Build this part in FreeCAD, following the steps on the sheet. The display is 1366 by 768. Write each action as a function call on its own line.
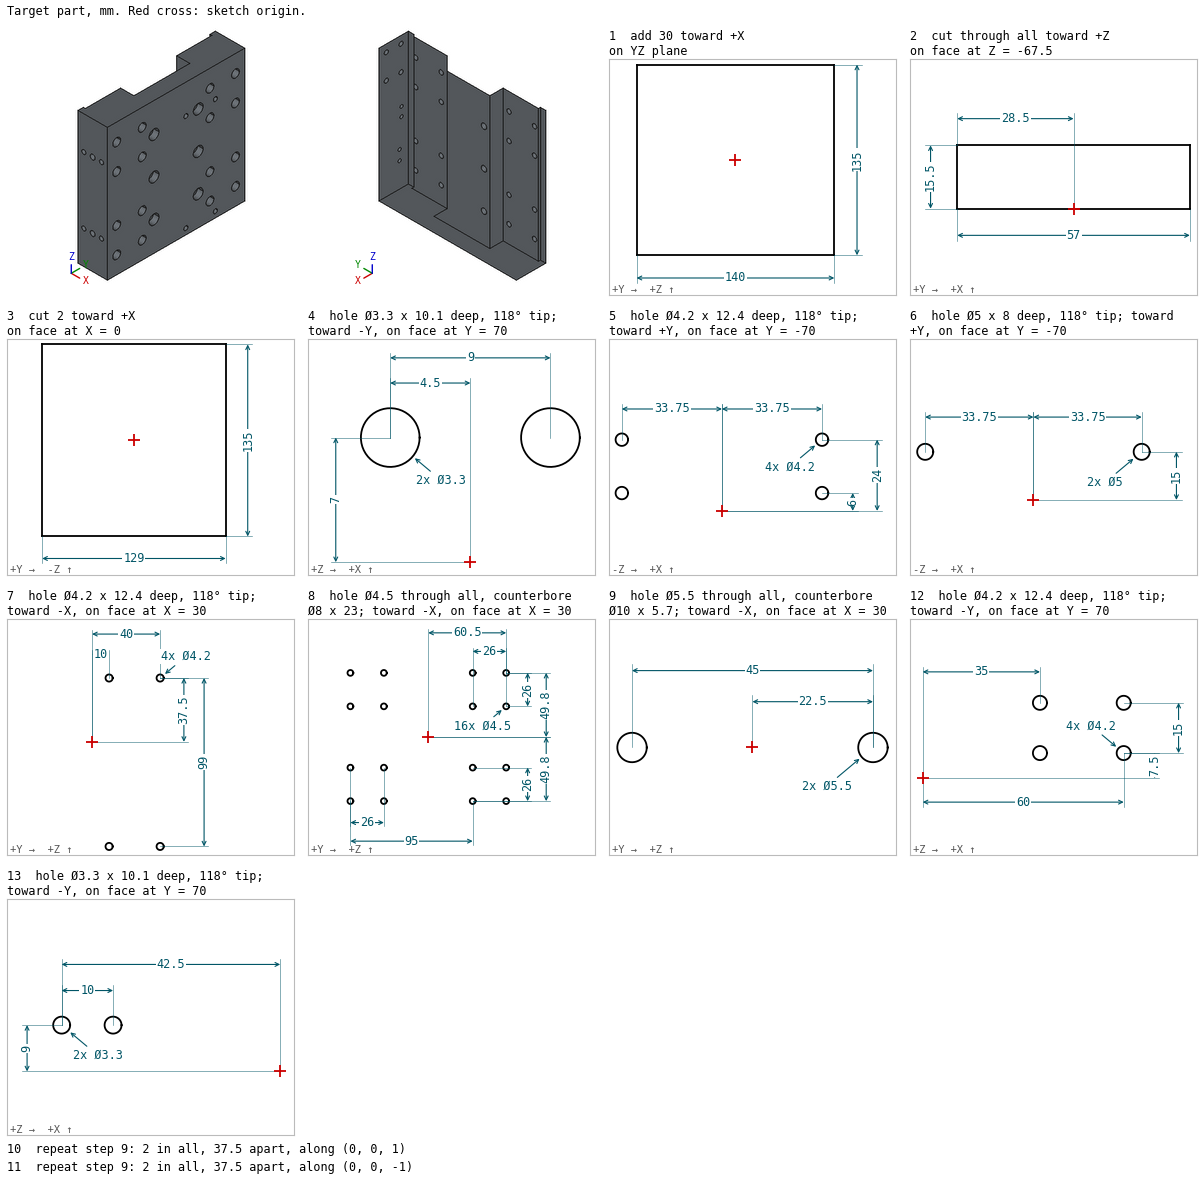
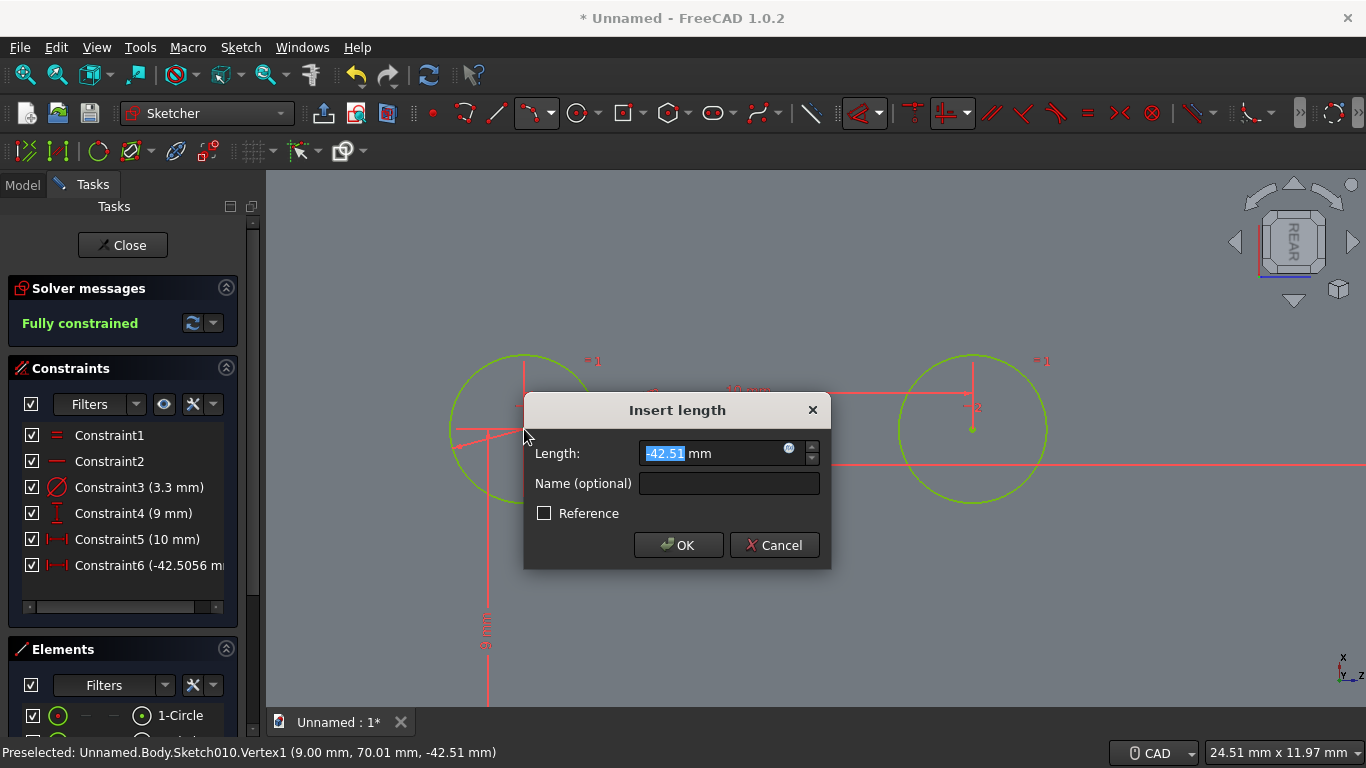
text(-42.5)
key(Return)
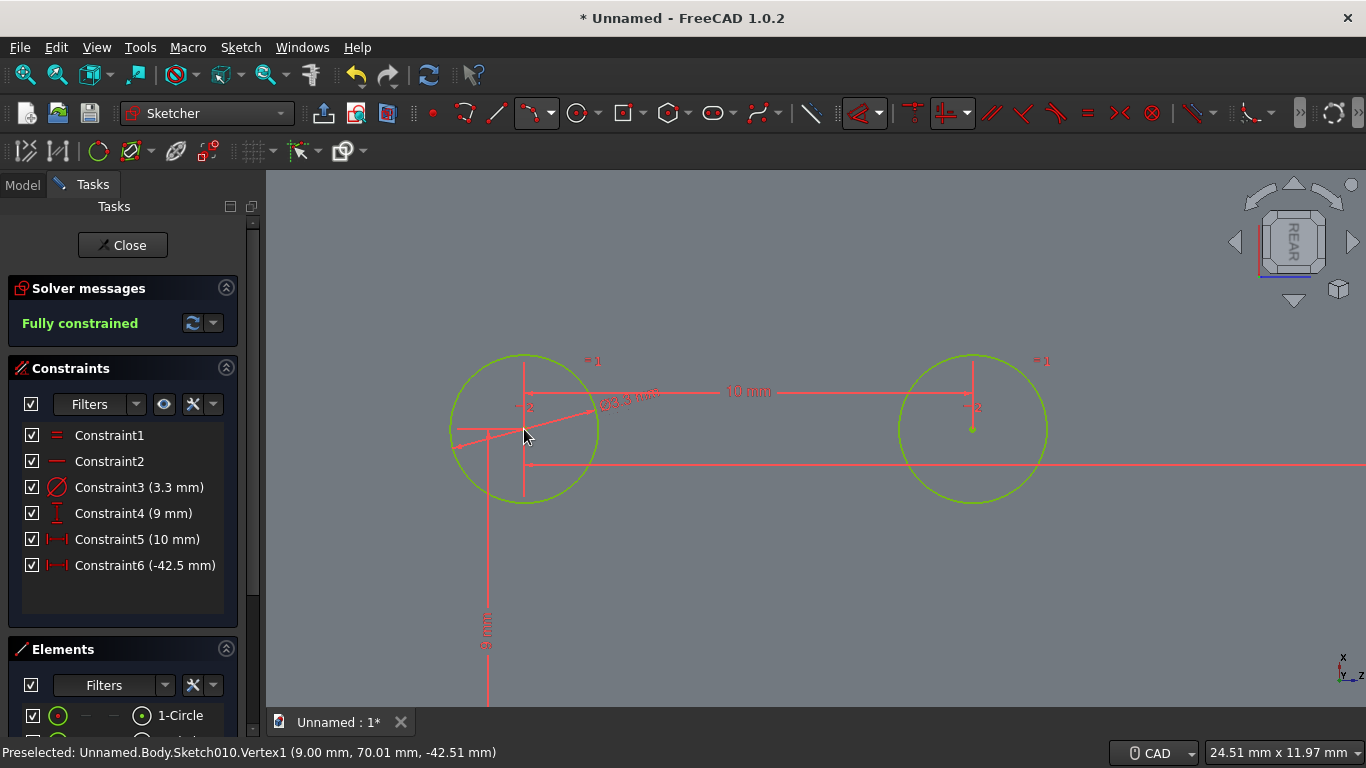
click(123, 245)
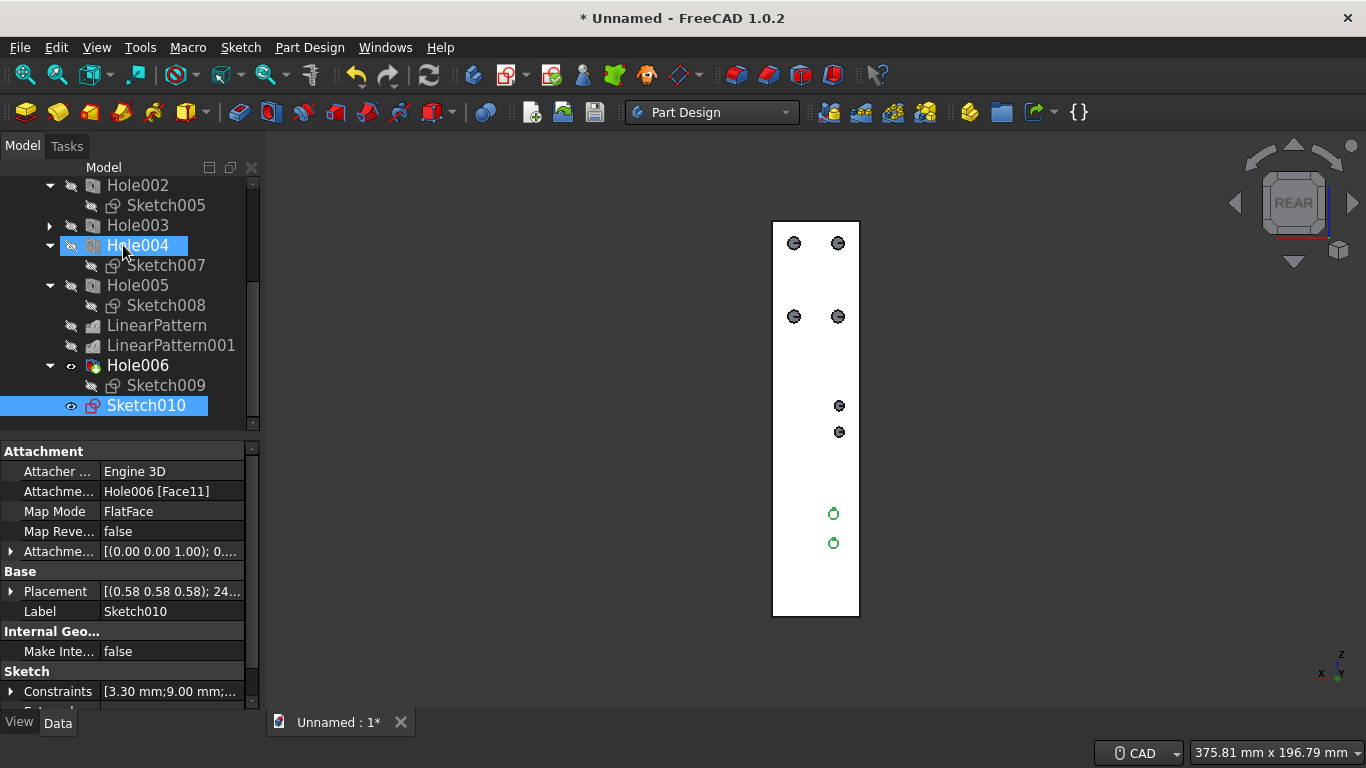
click(272, 112)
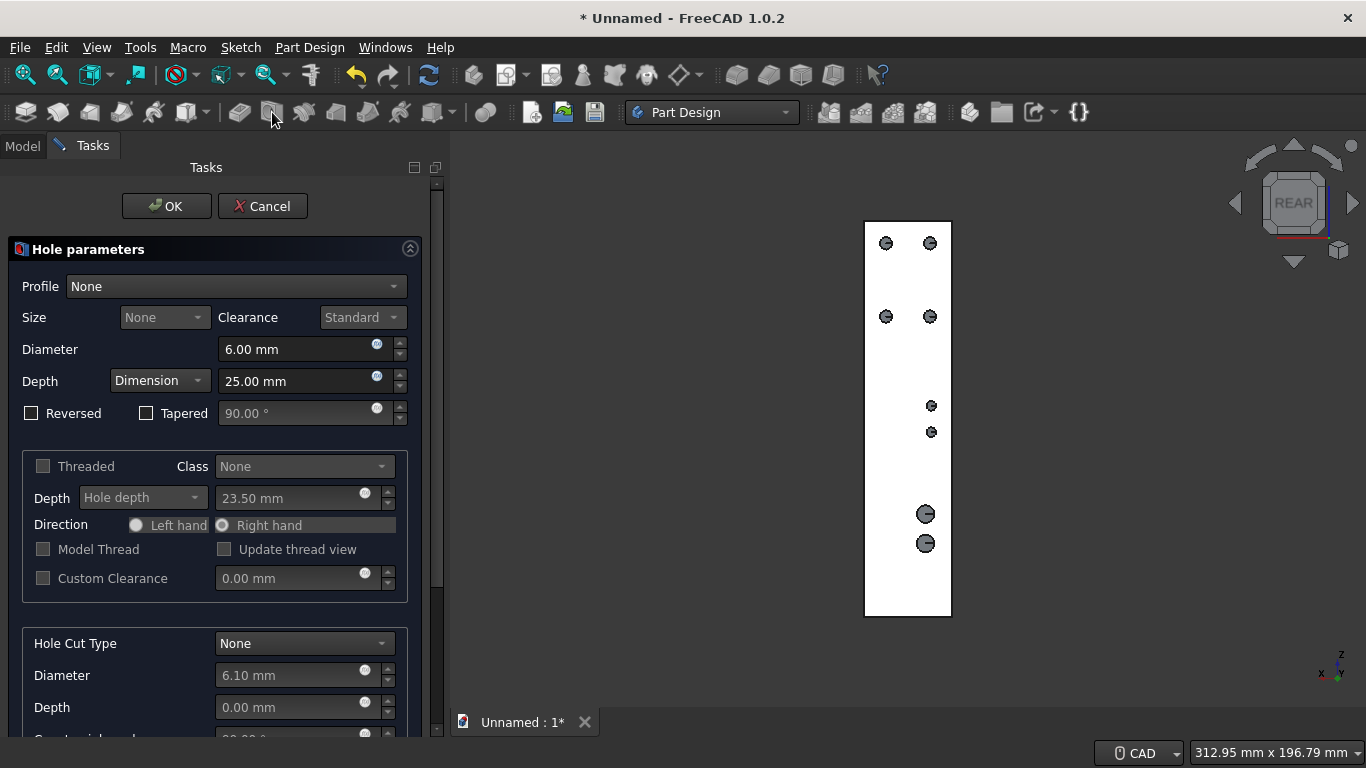
triple_click(305, 349)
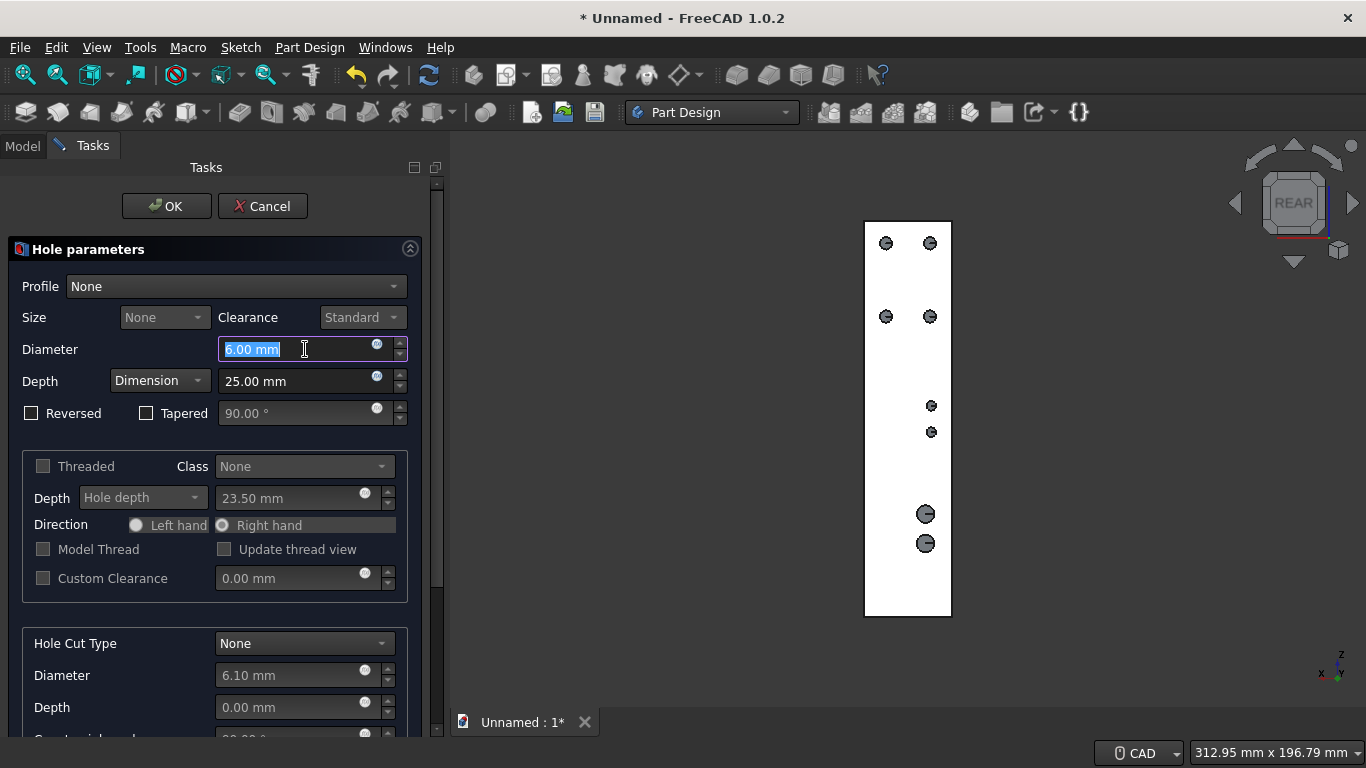
text(3.3)
key(Tab)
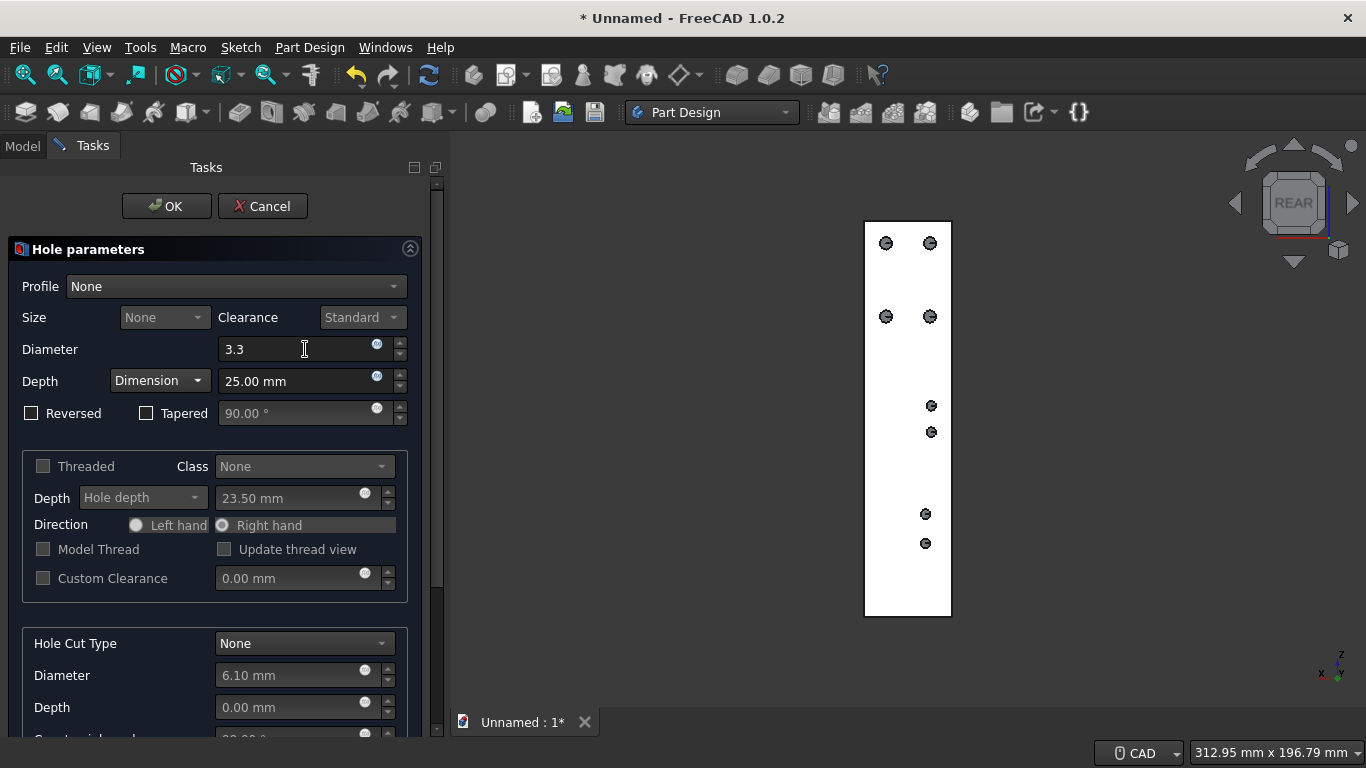
triple_click(305, 381)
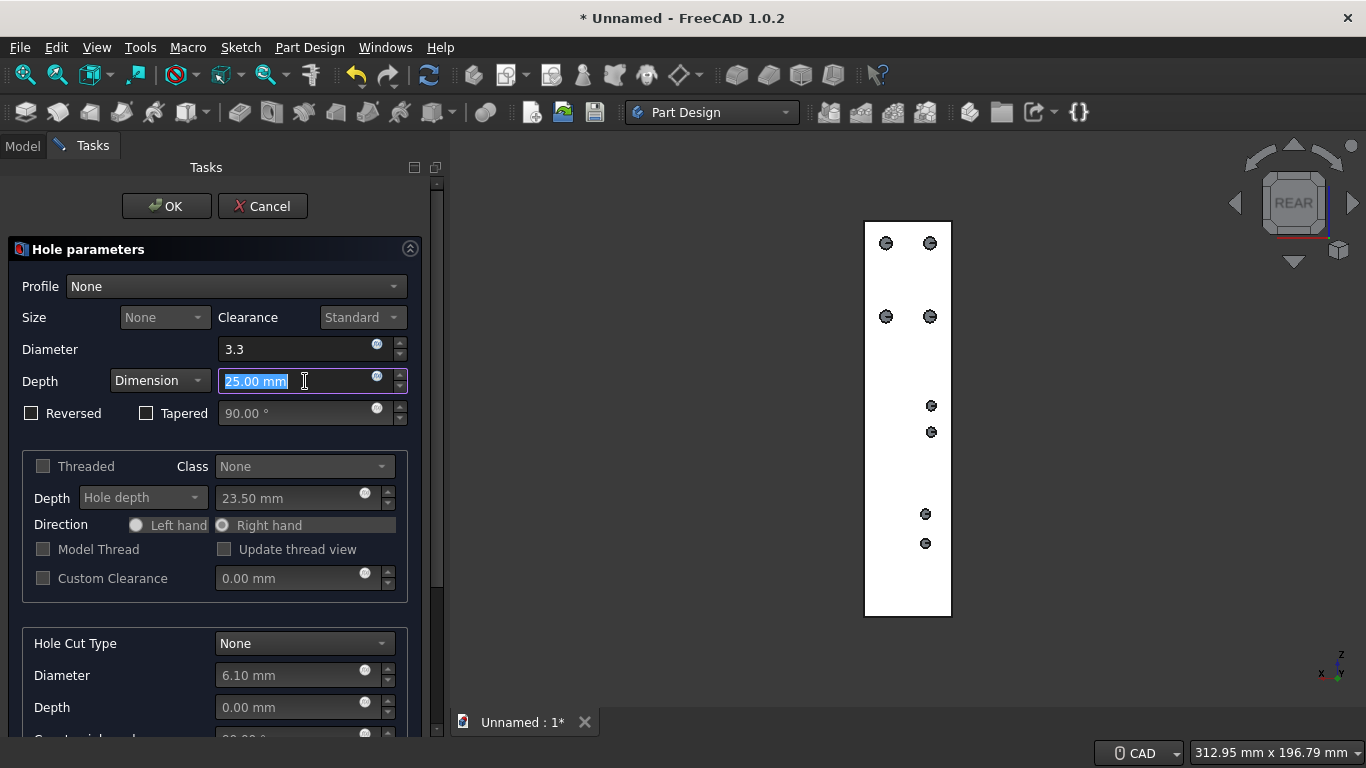
text(10.1)
key(Tab)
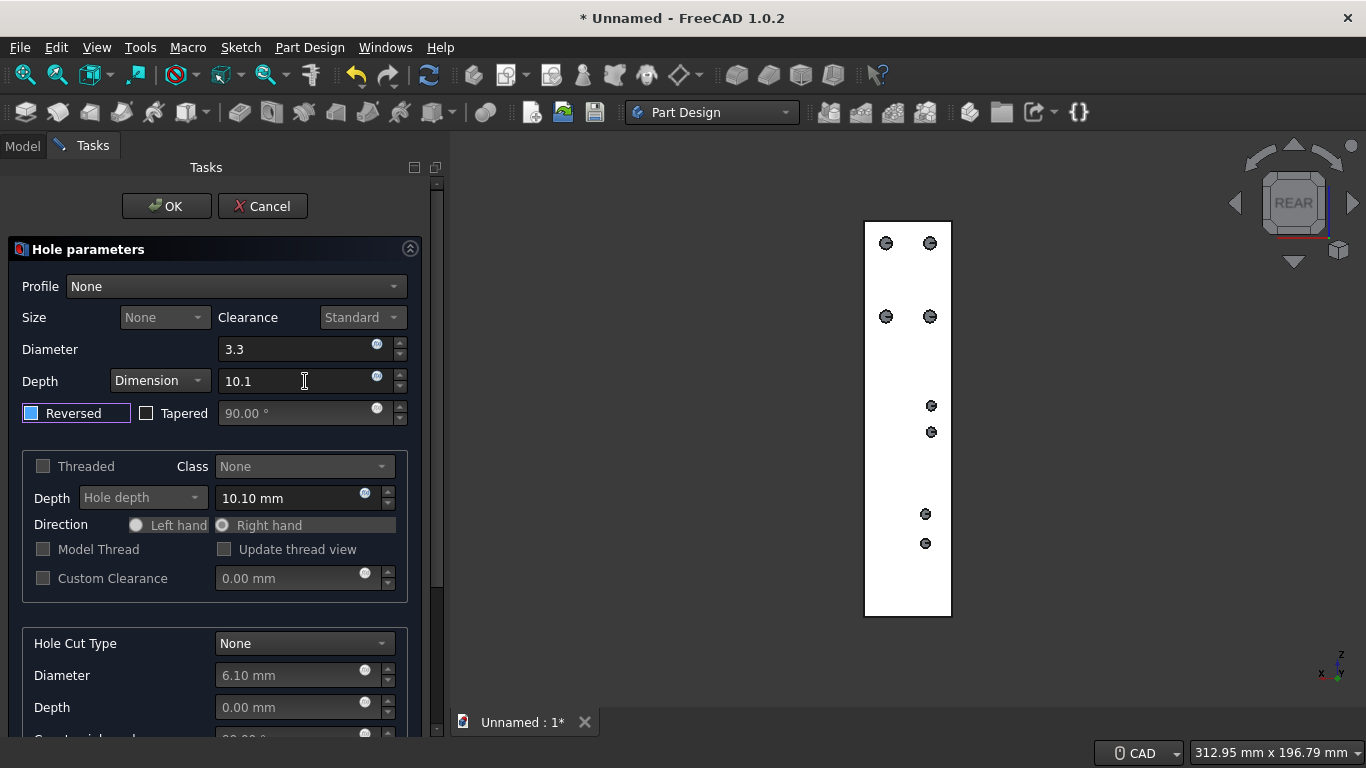
click(167, 206)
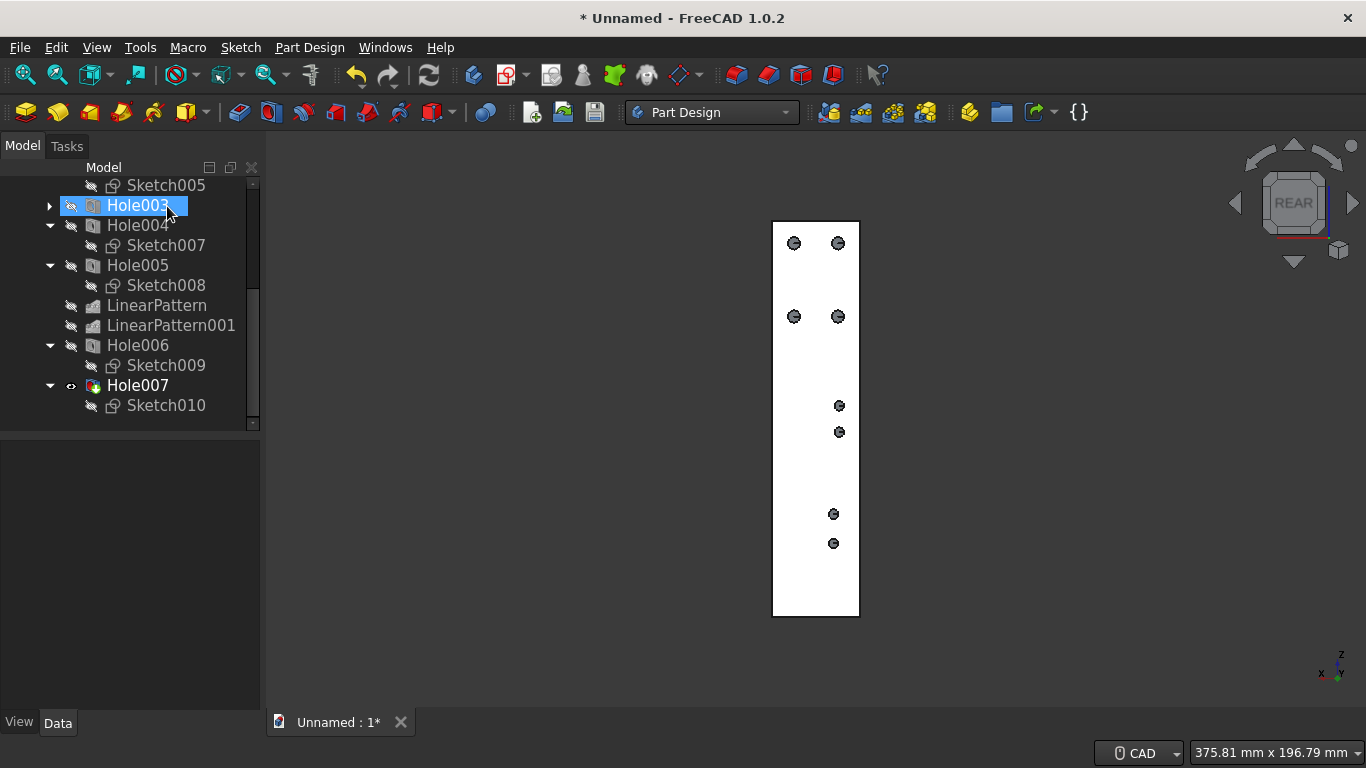
key(0)